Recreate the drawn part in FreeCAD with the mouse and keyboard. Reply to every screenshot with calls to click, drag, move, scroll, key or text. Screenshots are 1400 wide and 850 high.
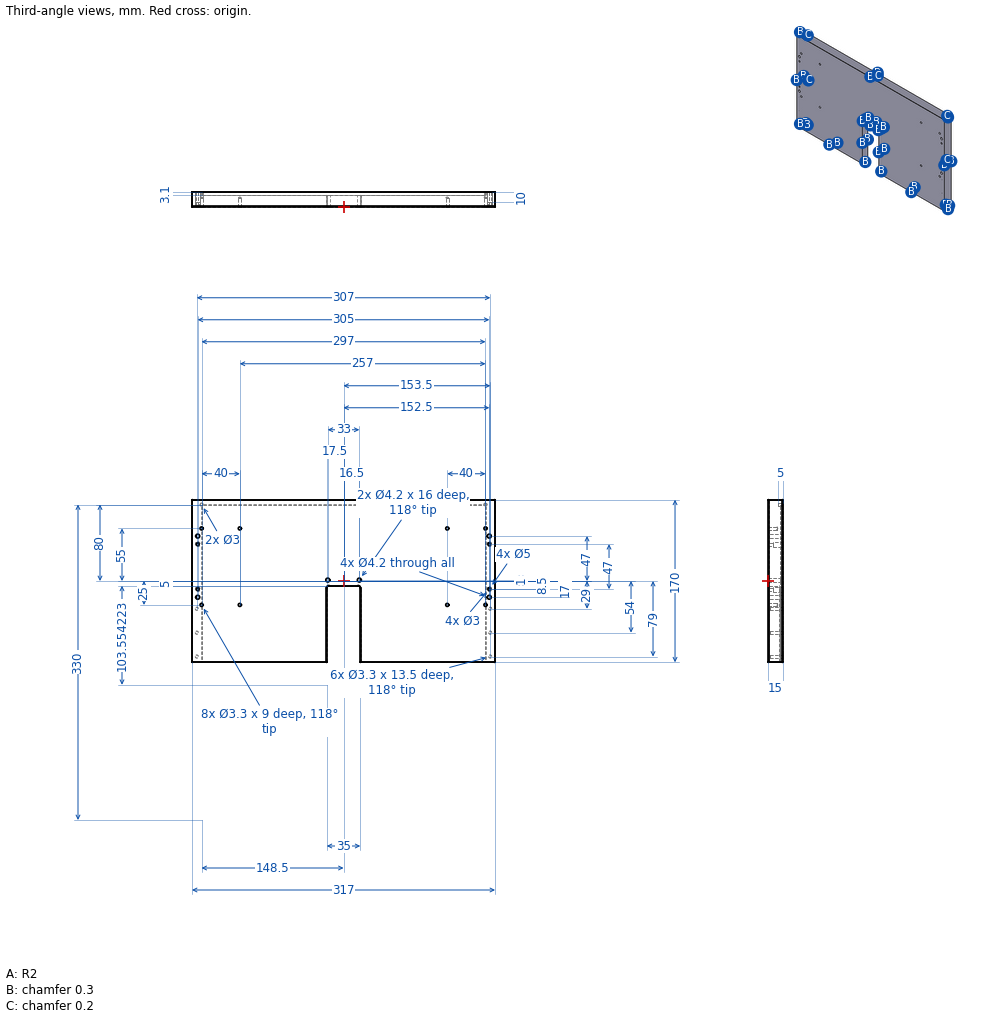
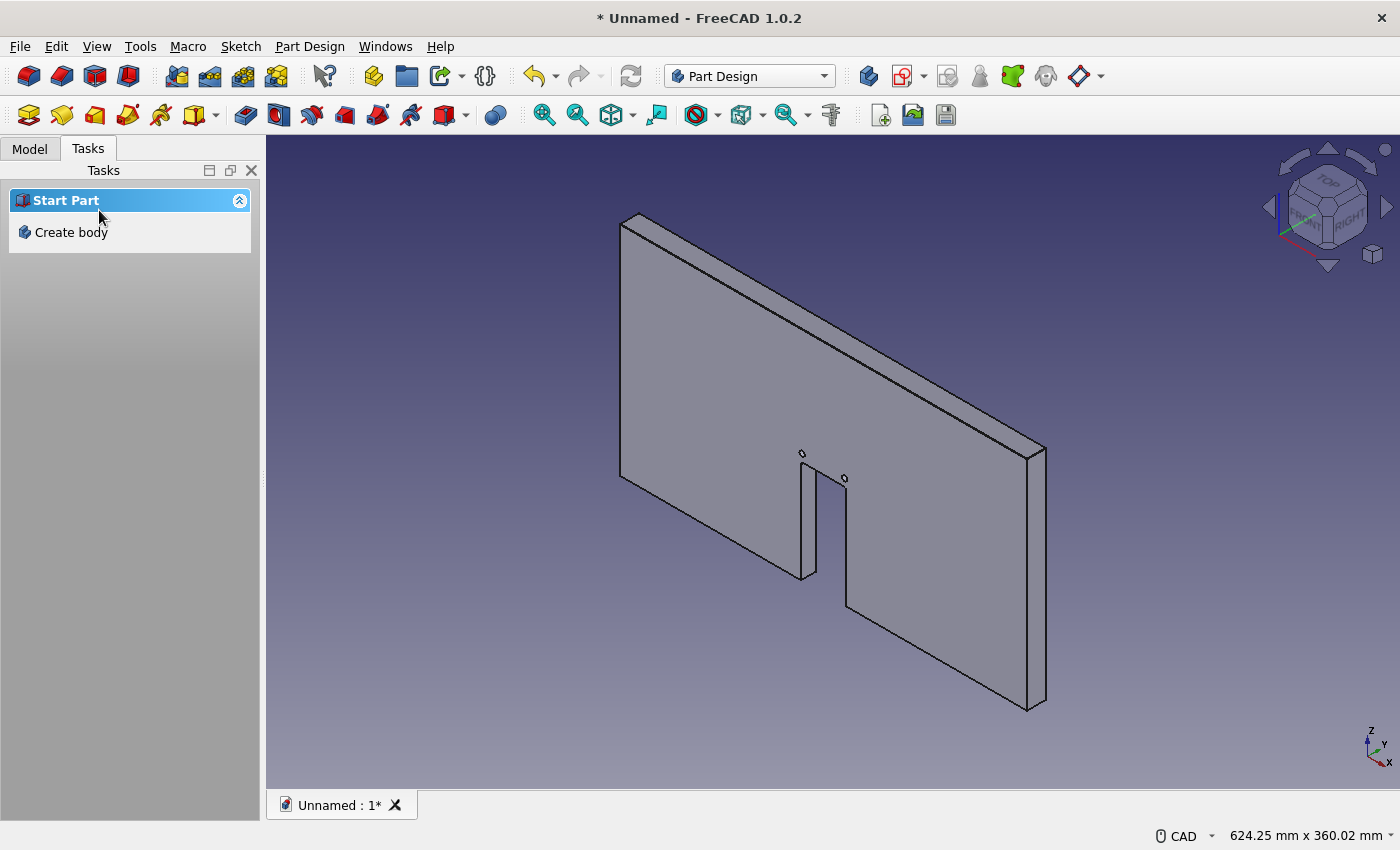
key(4)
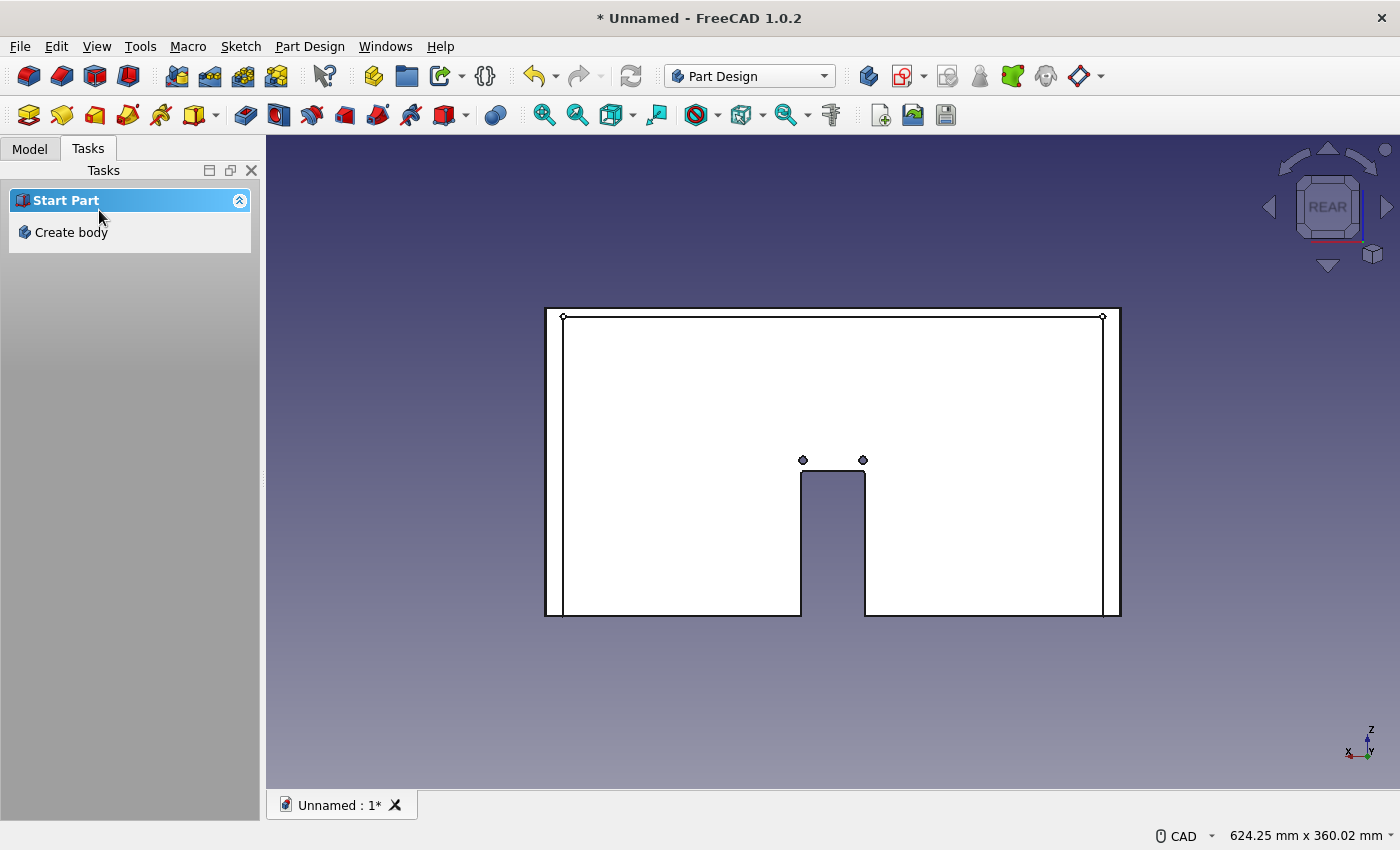
scroll(1110, 417, up, 3)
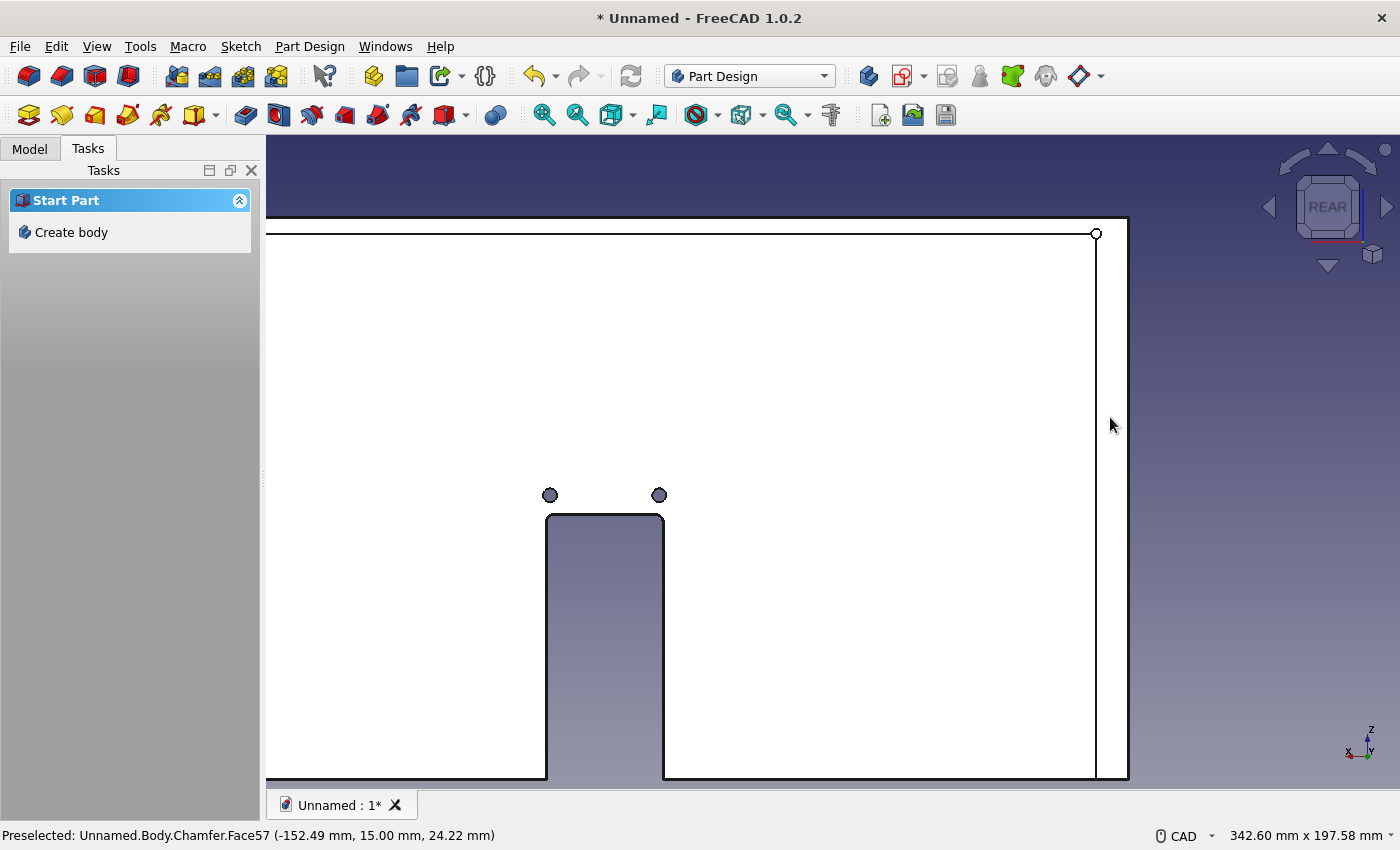
click(1109, 417)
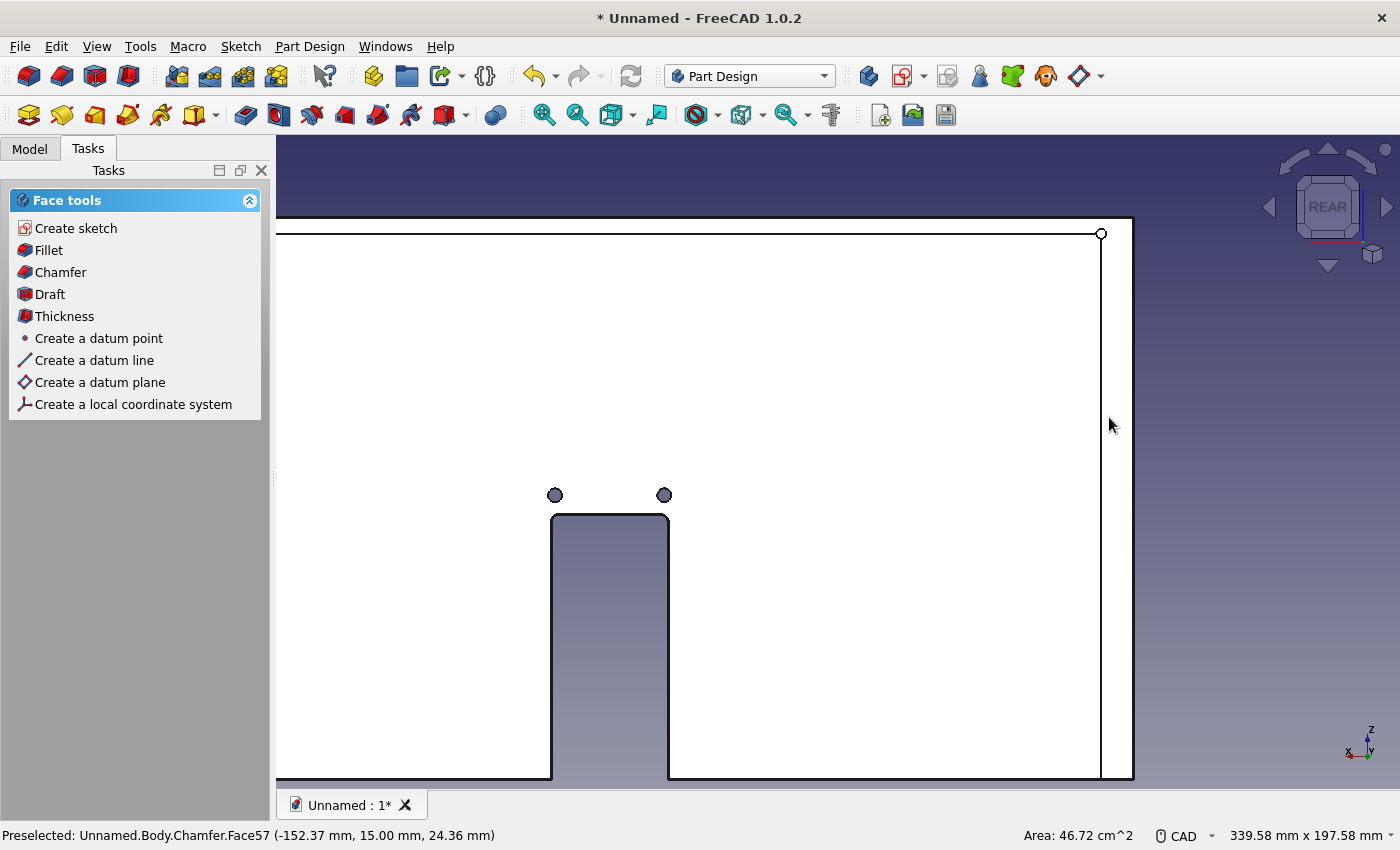
click(902, 76)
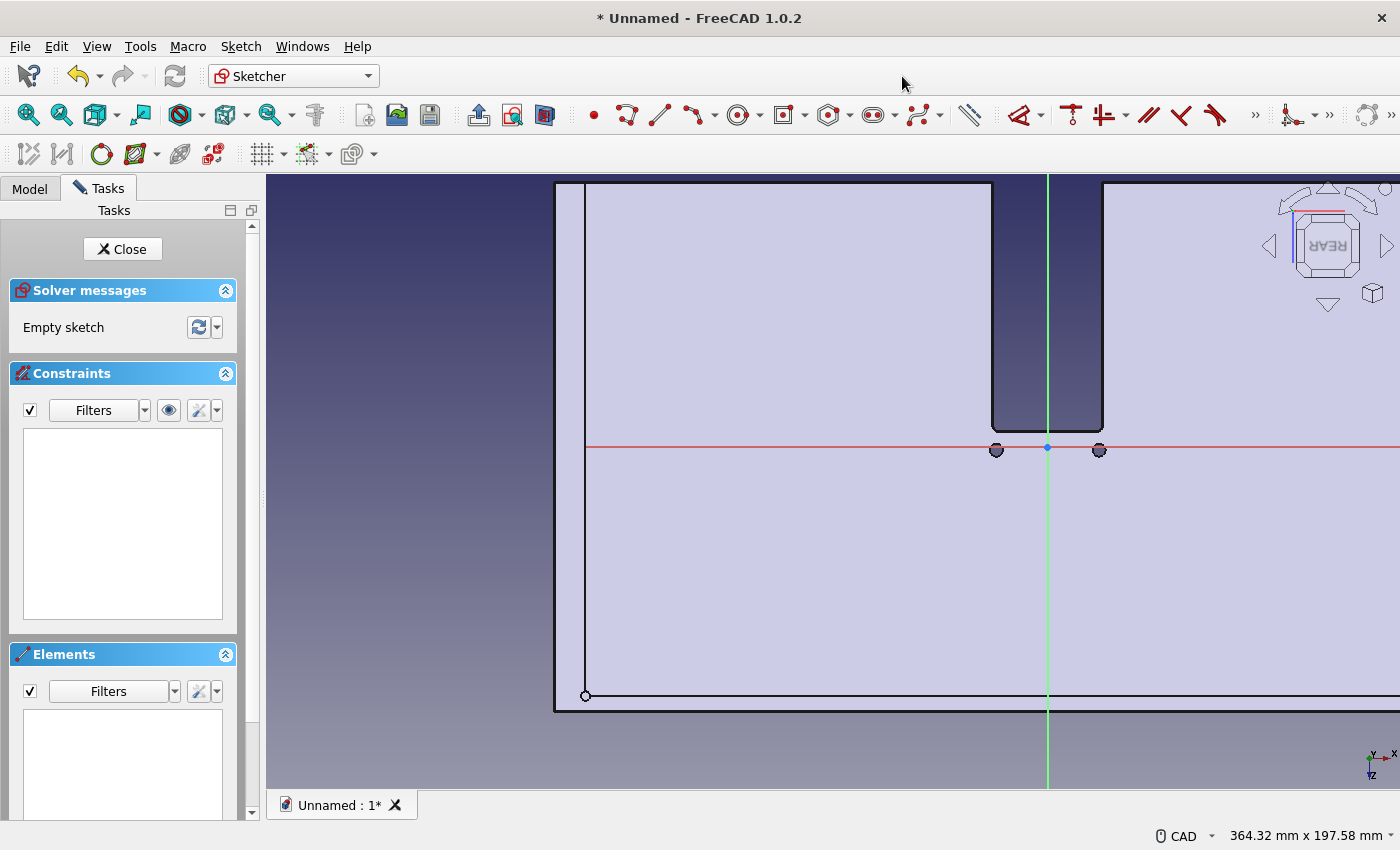
scroll(294, 457, down, 2)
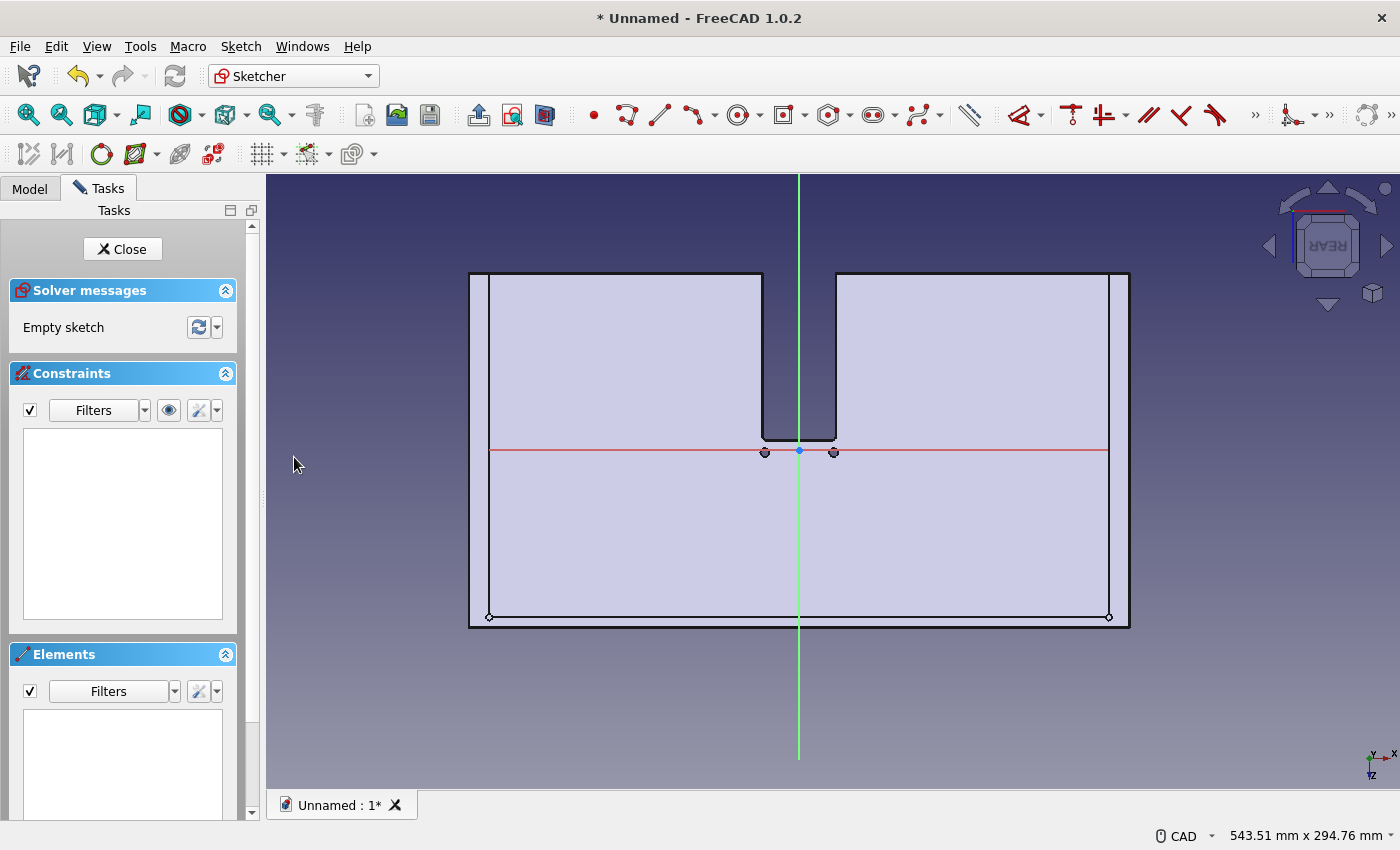
click(738, 116)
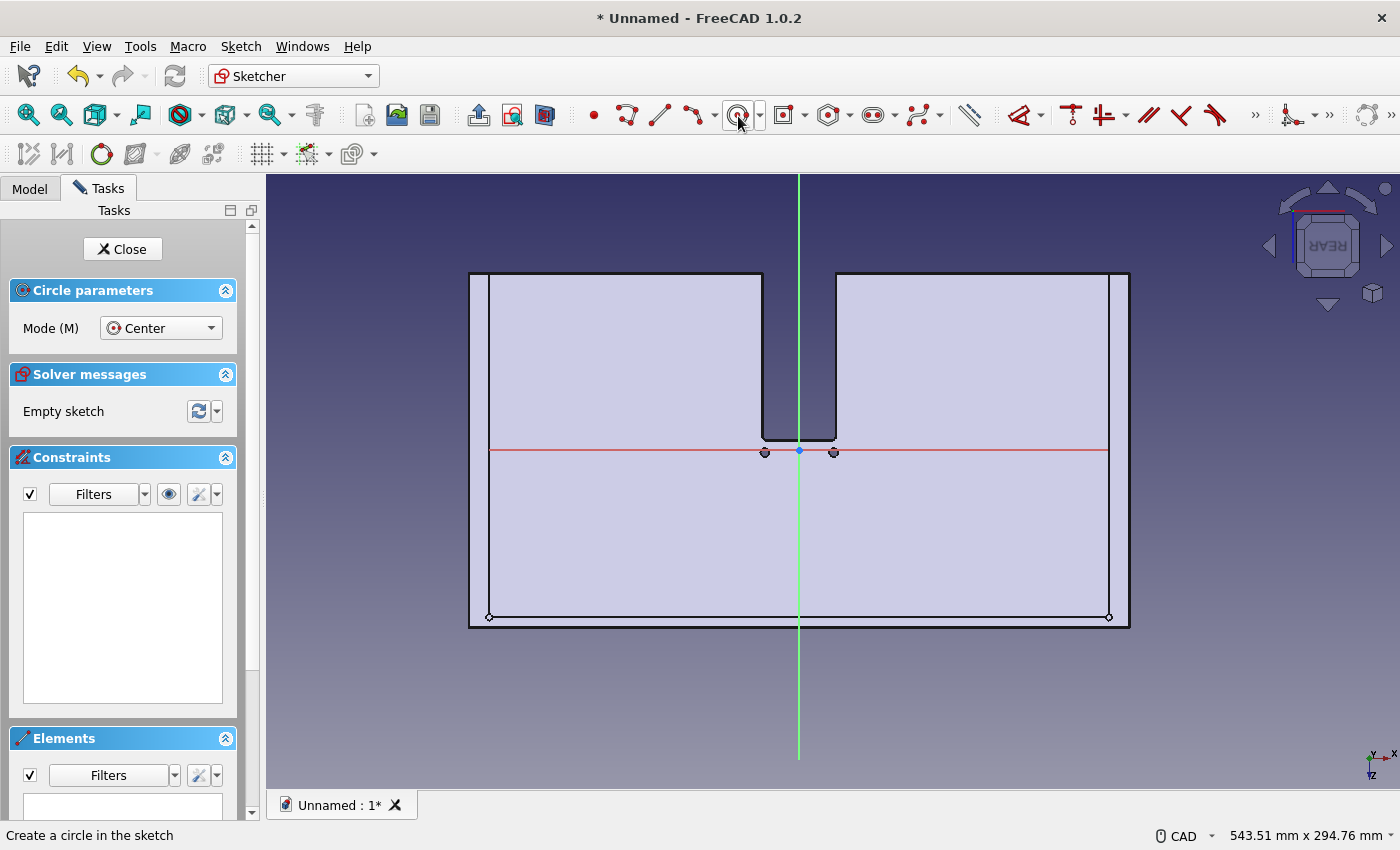
scroll(1117, 415, up, 9)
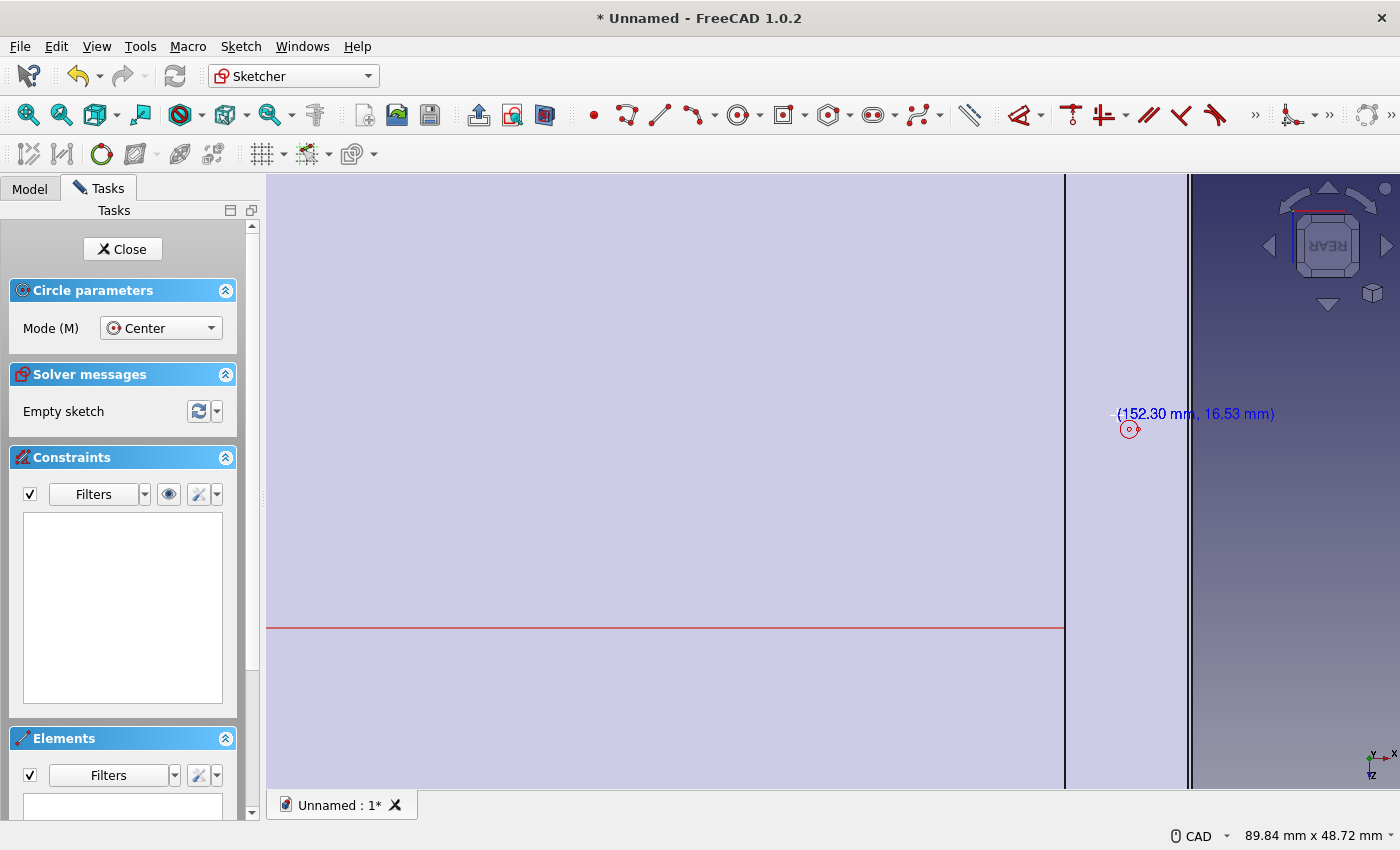
scroll(1076, 415, down, 9)